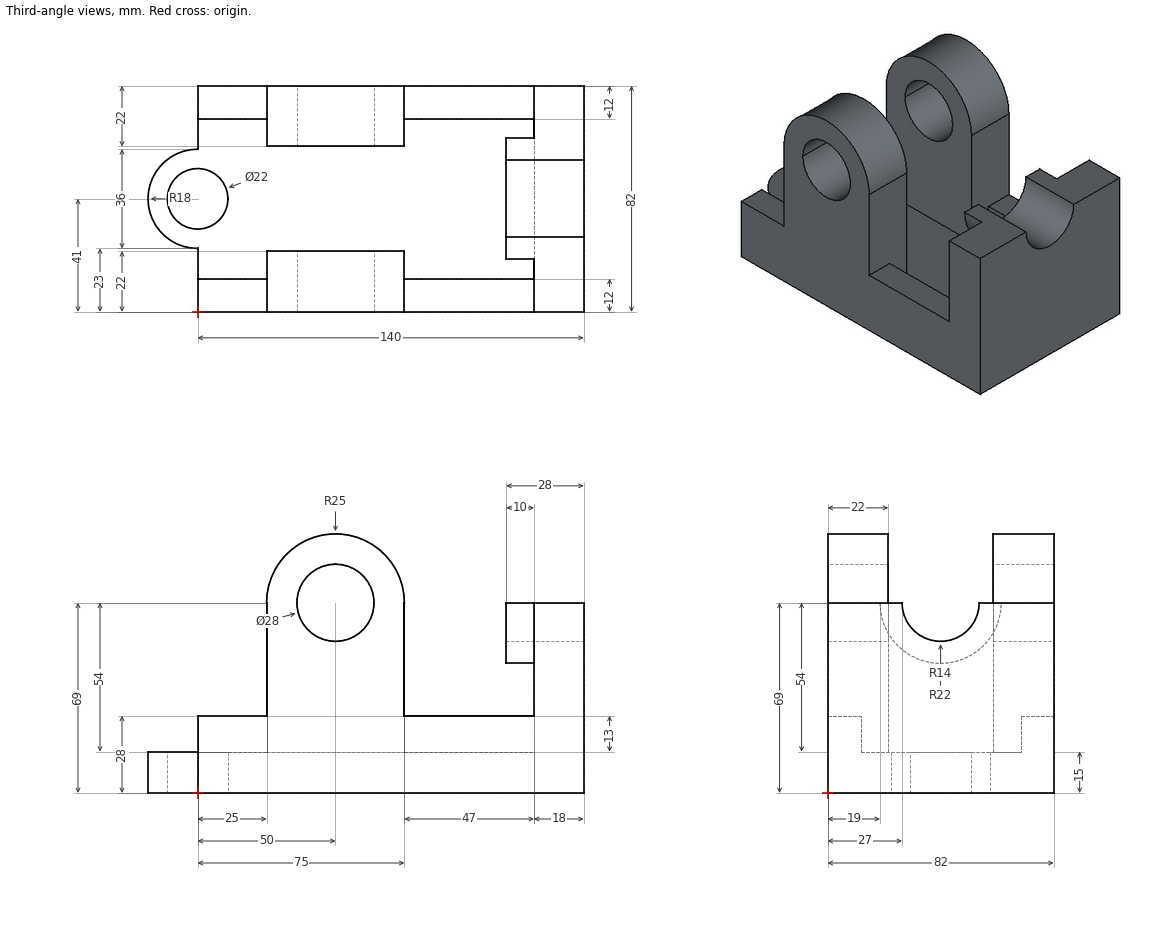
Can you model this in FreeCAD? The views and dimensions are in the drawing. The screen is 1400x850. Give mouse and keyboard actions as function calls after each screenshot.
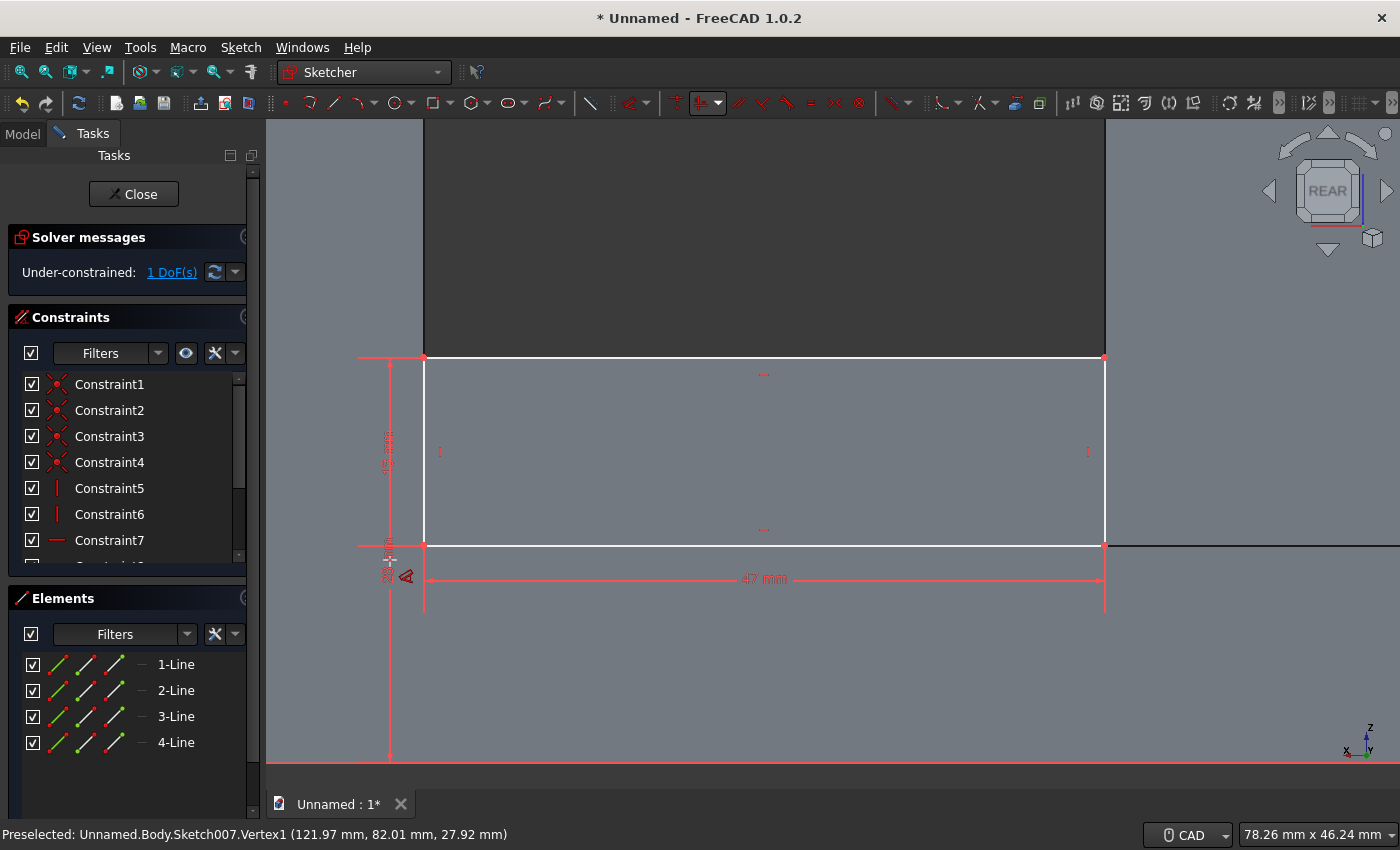
click(1105, 546)
click(1170, 512)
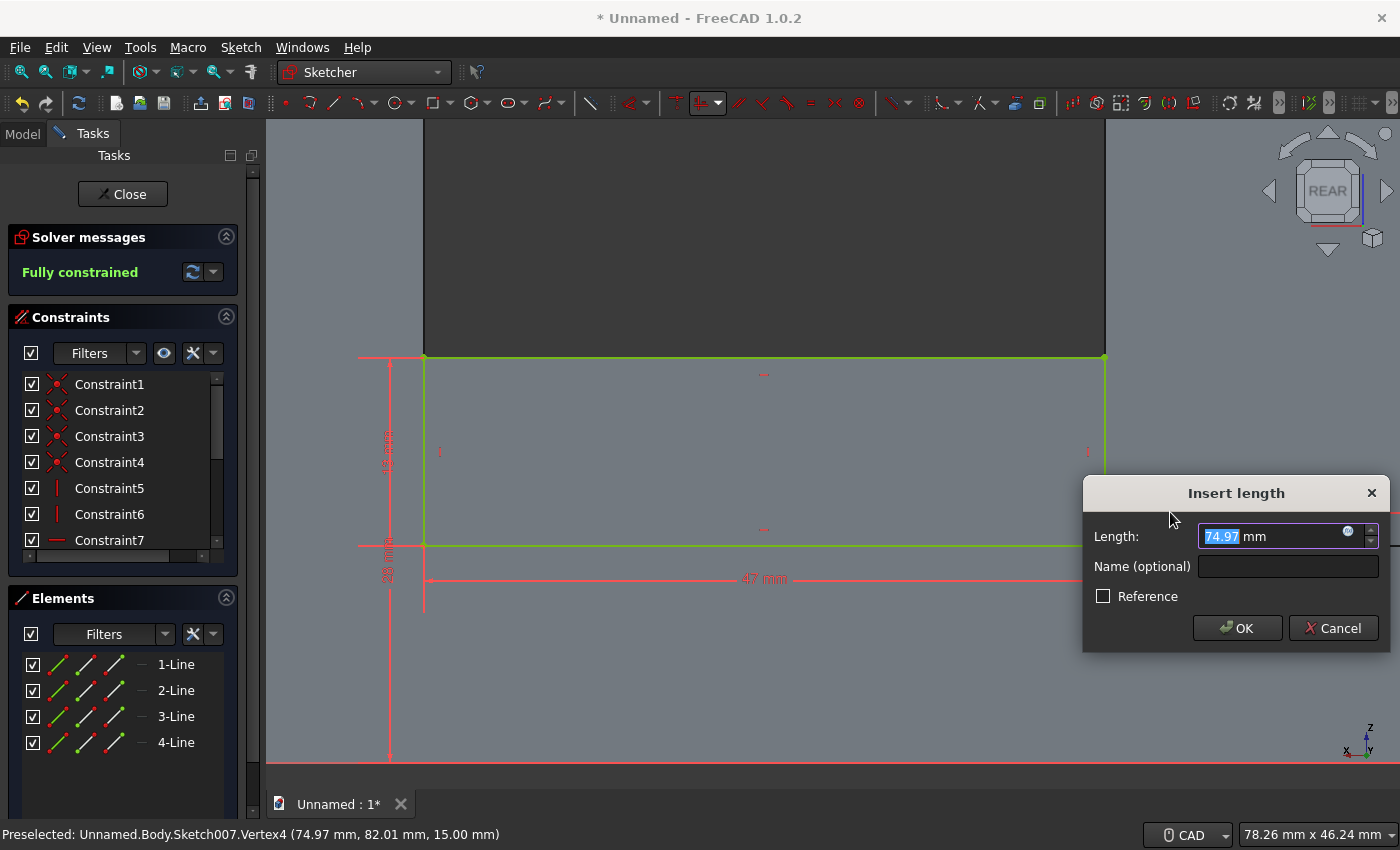
text(75)
key(Return)
key(Escape)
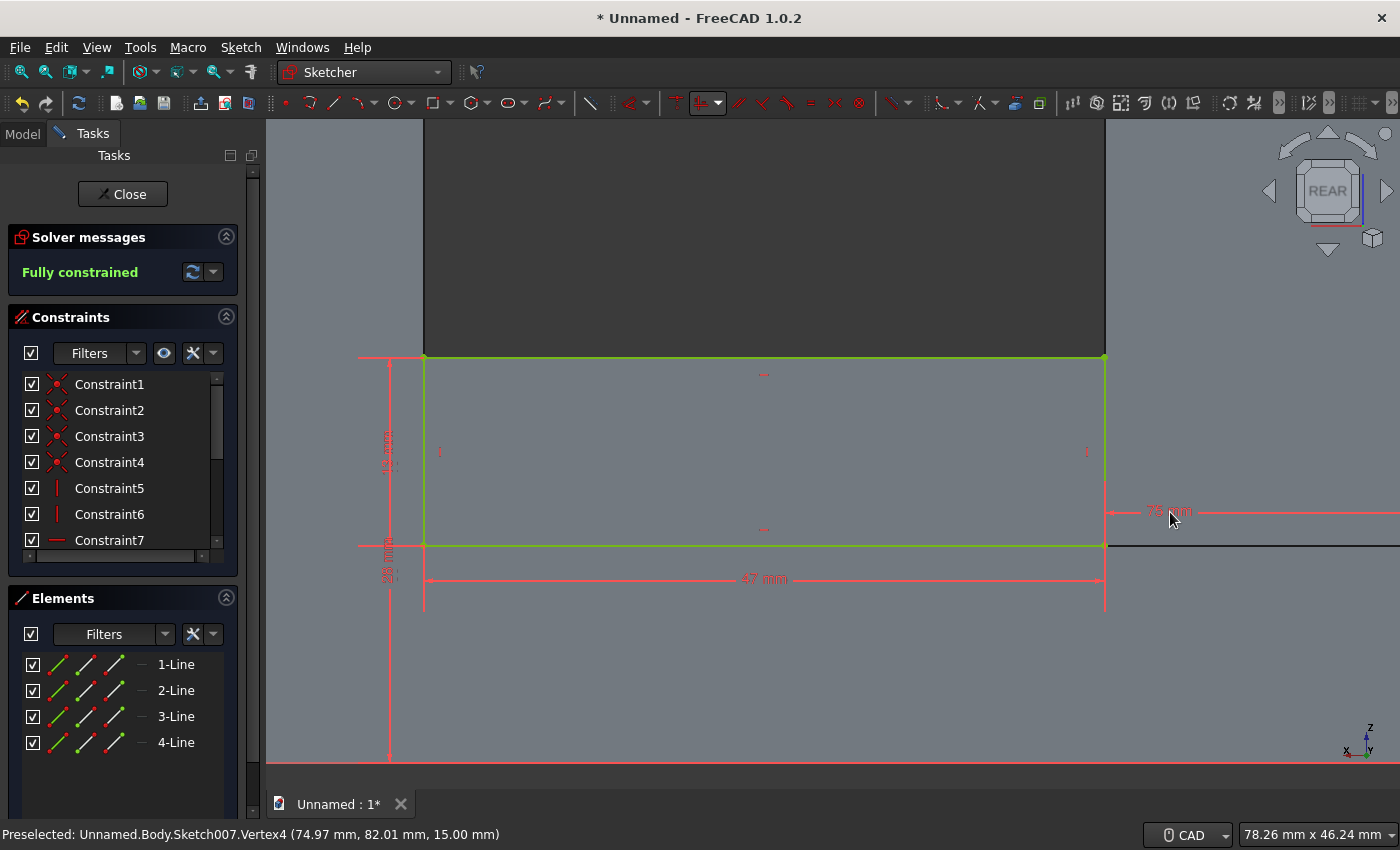
click(123, 194)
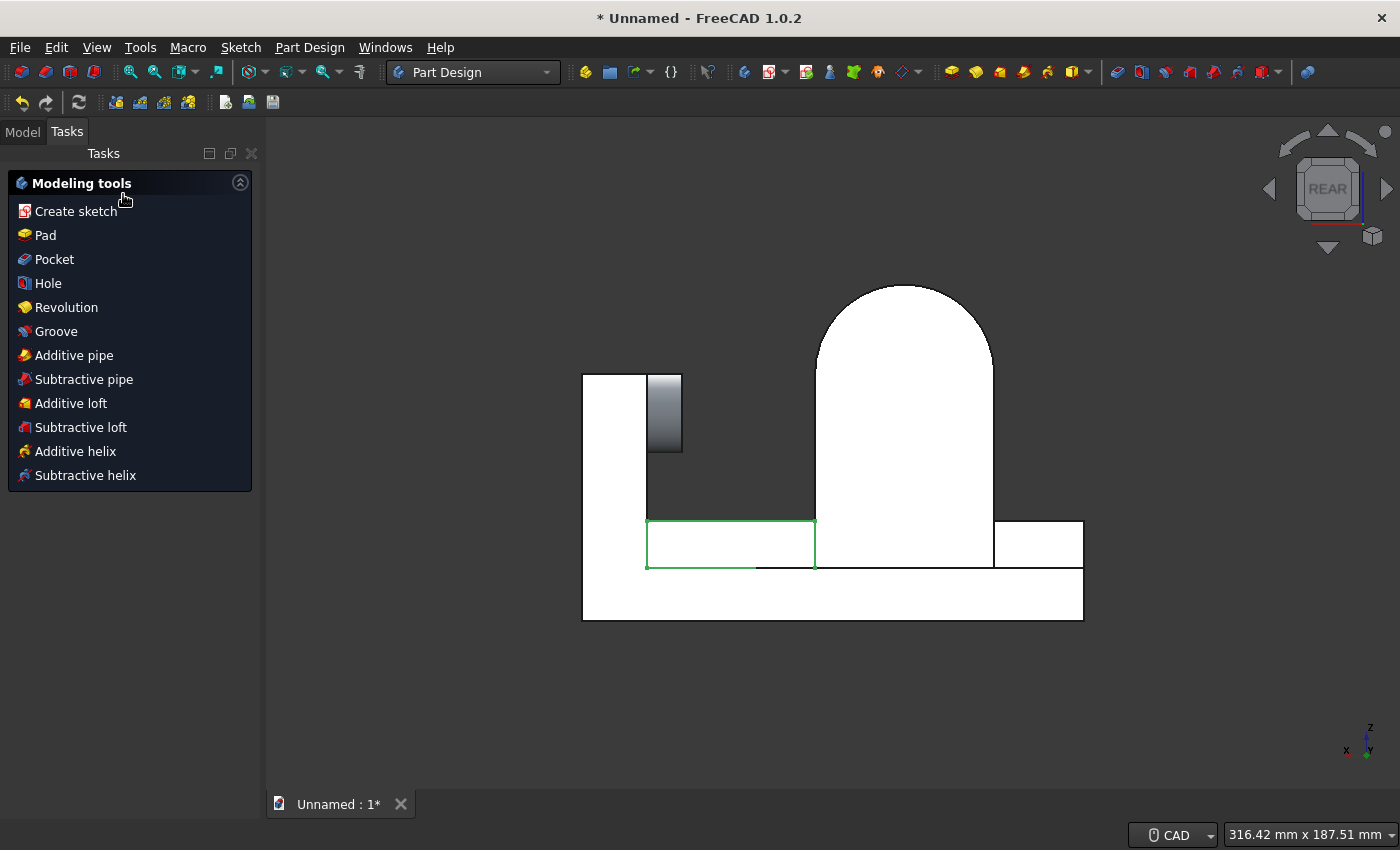
click(952, 72)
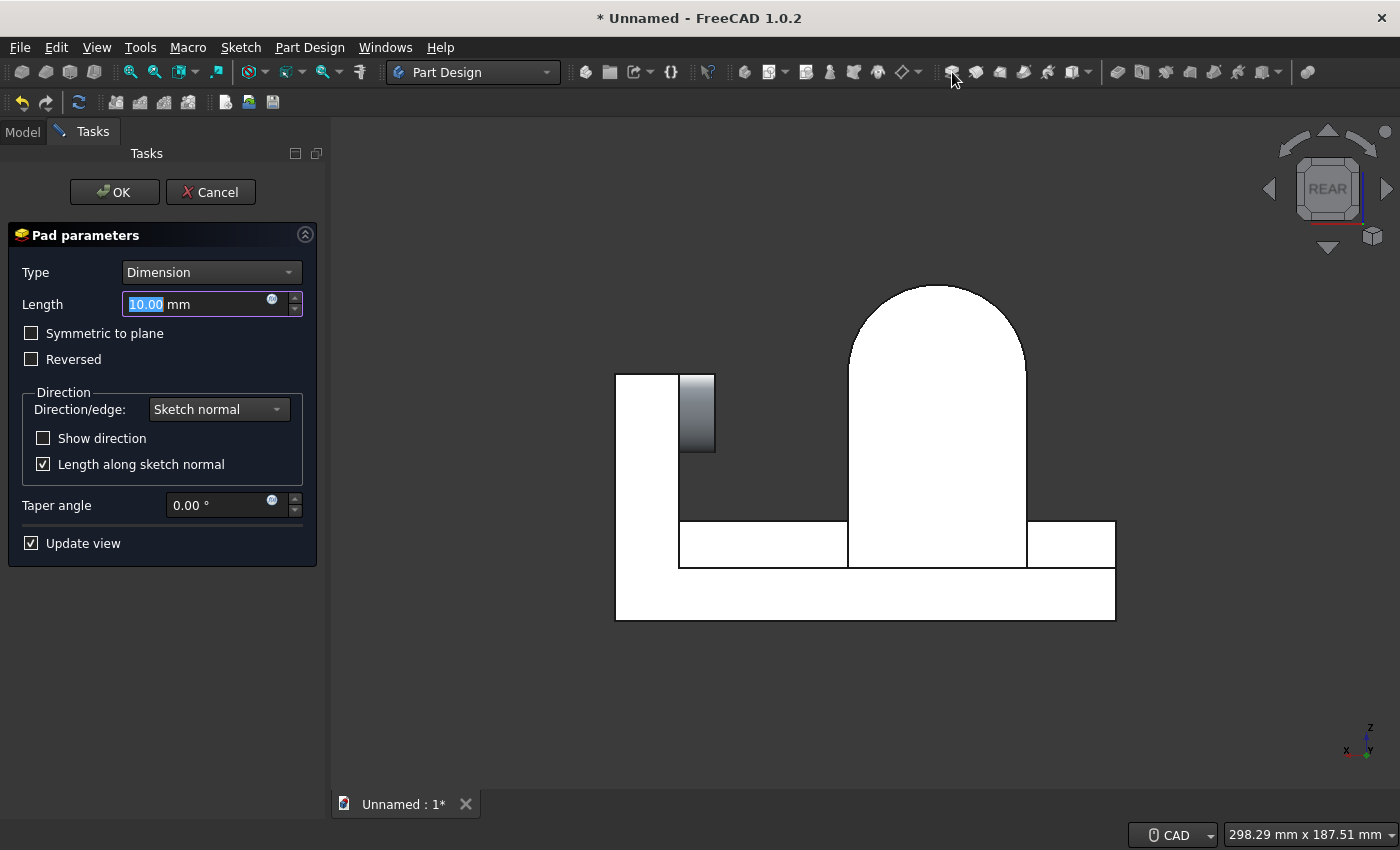
text(12)
key(Tab)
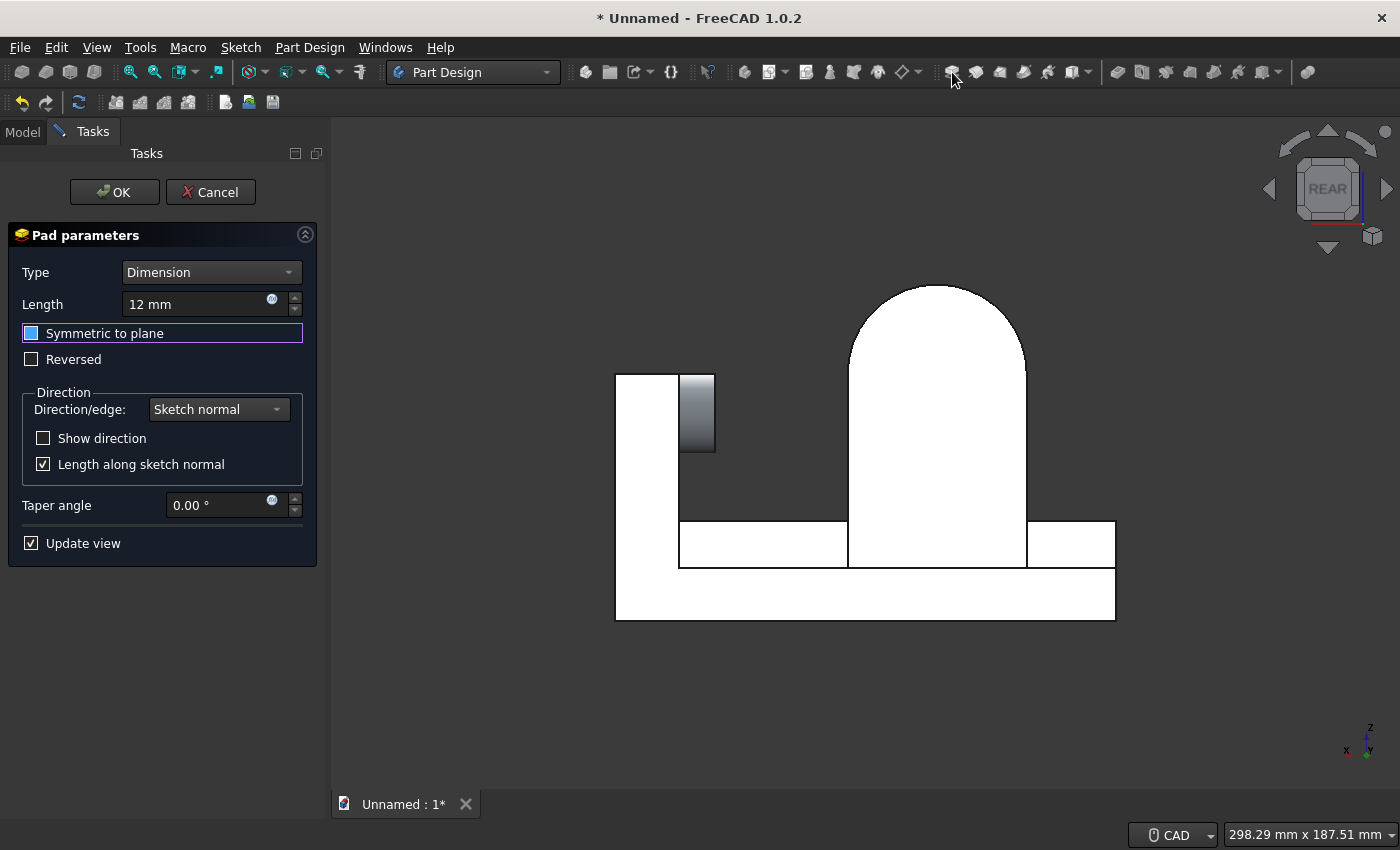
click(30, 359)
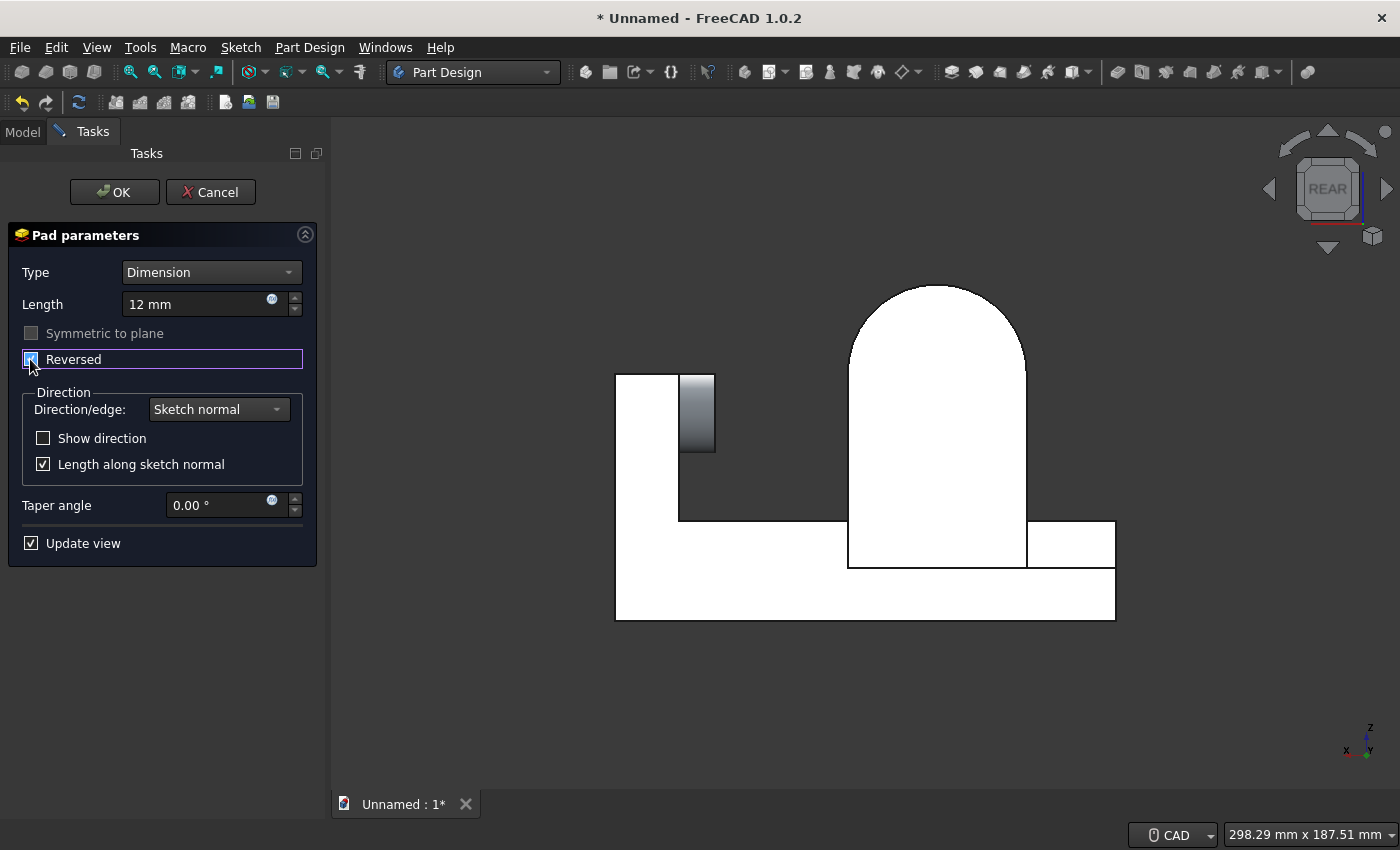
click(115, 192)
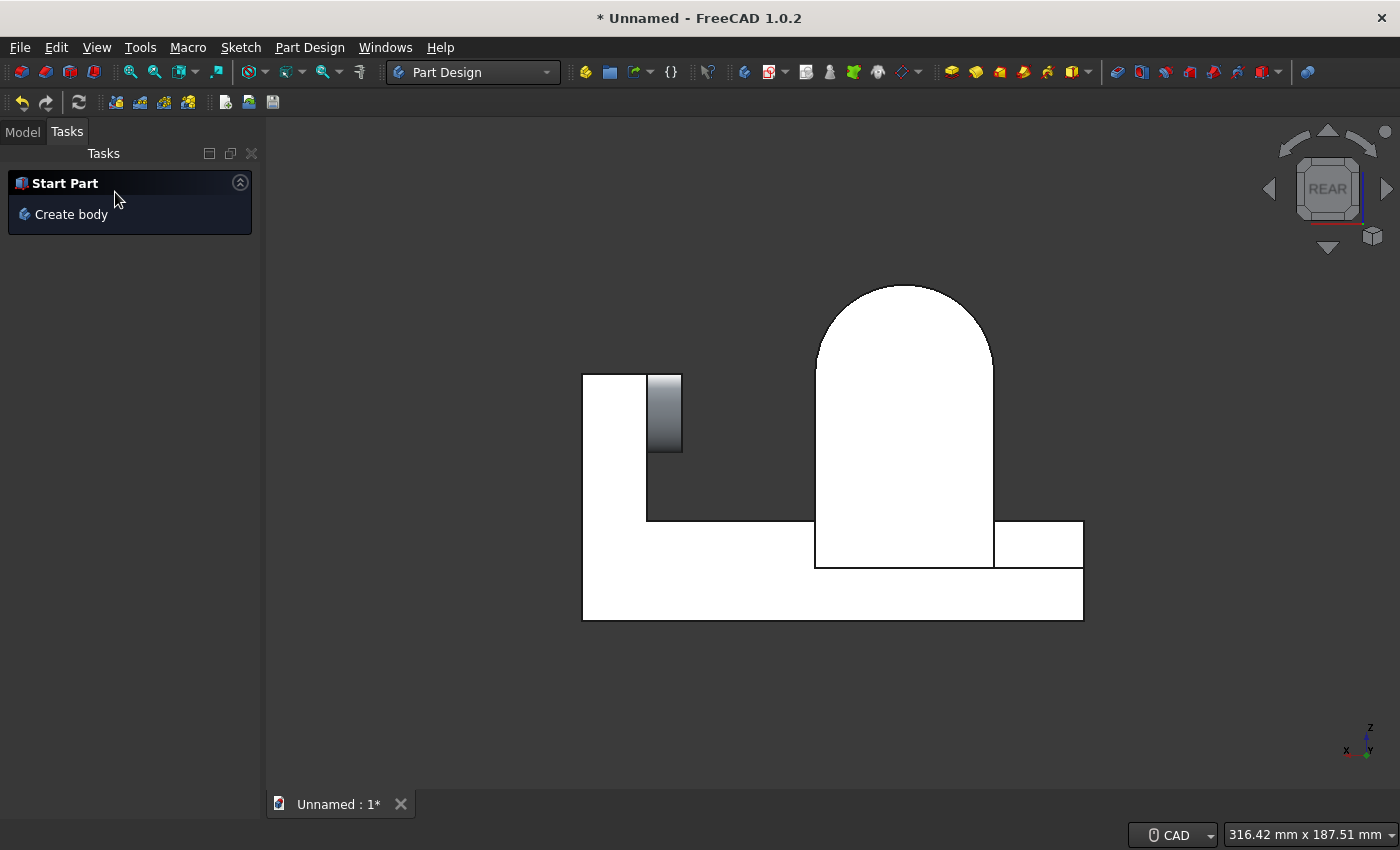
click(23, 131)